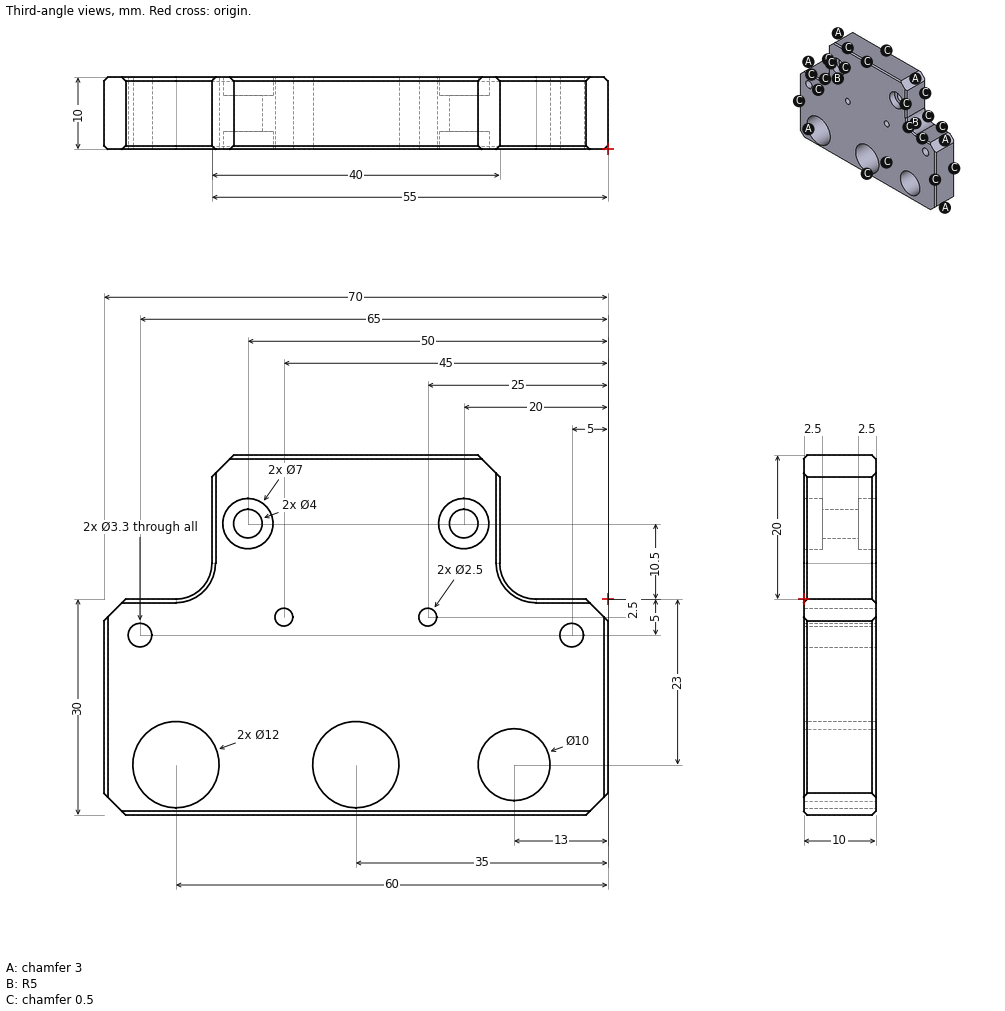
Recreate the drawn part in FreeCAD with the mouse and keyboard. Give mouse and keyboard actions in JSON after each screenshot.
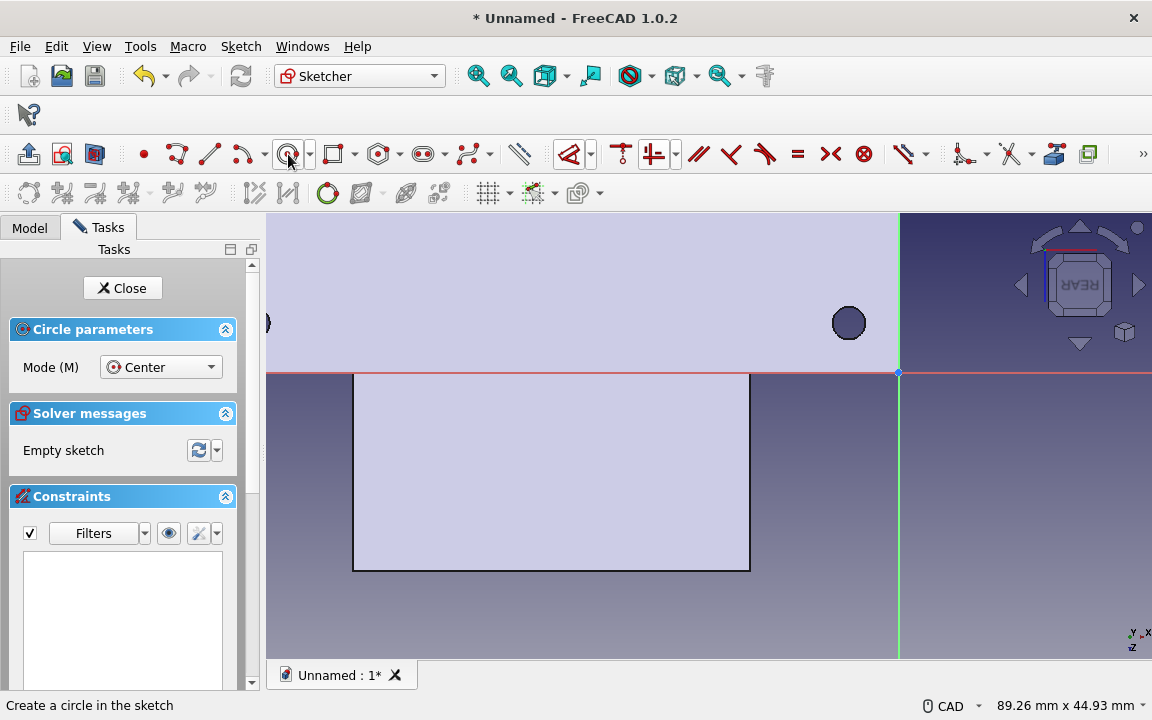
{"action": "left_click", "coordinate": [402, 477]}
{"action": "left_click", "coordinate": [416, 463]}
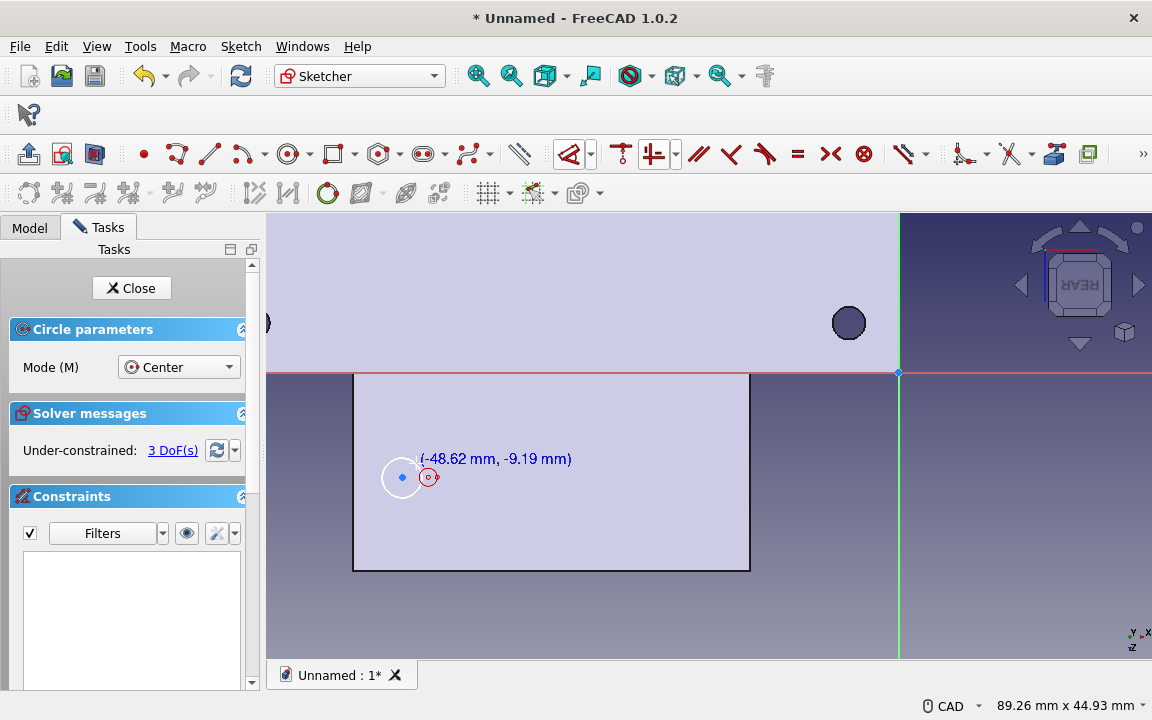
{"action": "left_click", "coordinate": [700, 477]}
{"action": "left_click", "coordinate": [714, 463]}
{"action": "key", "text": "Escape"}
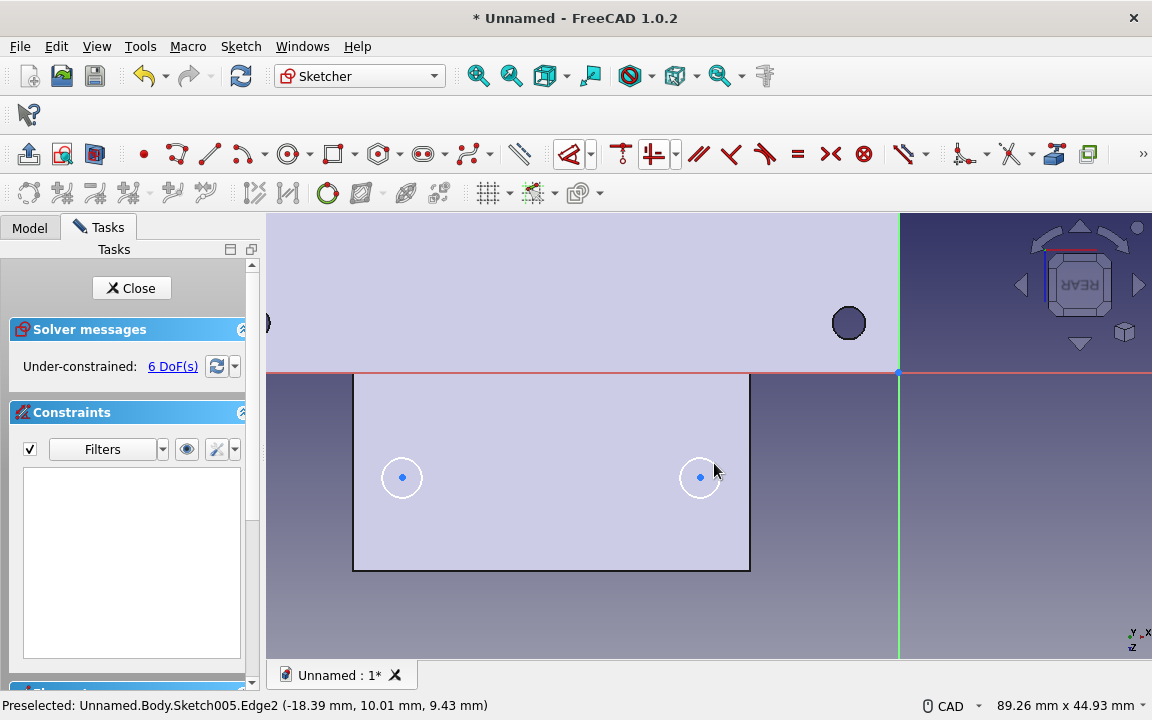
{"action": "left_click", "coordinate": [416, 464]}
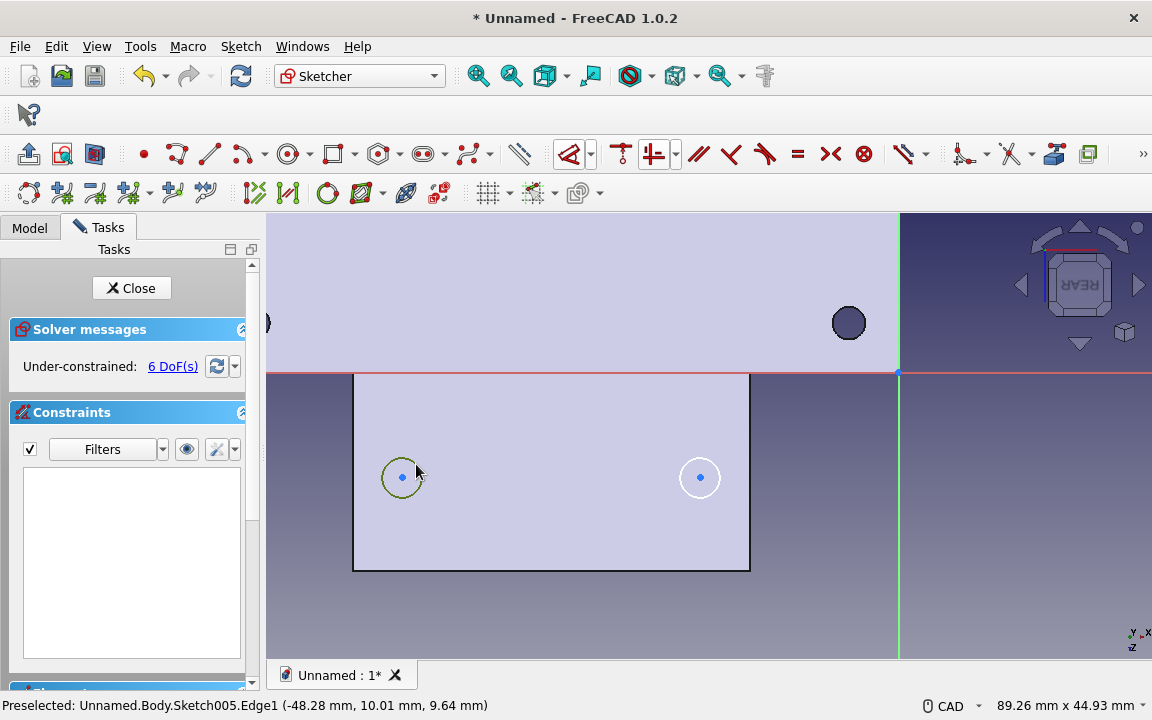
{"action": "left_click", "coordinate": [714, 464]}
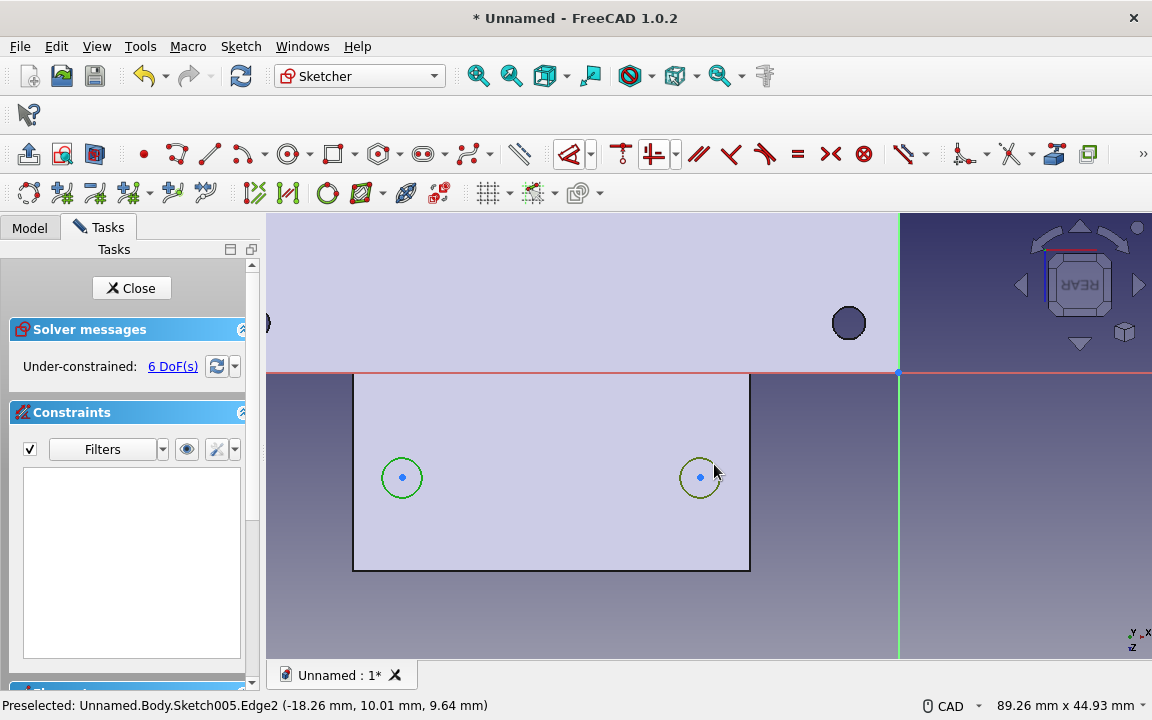
{"action": "left_click", "coordinate": [798, 154]}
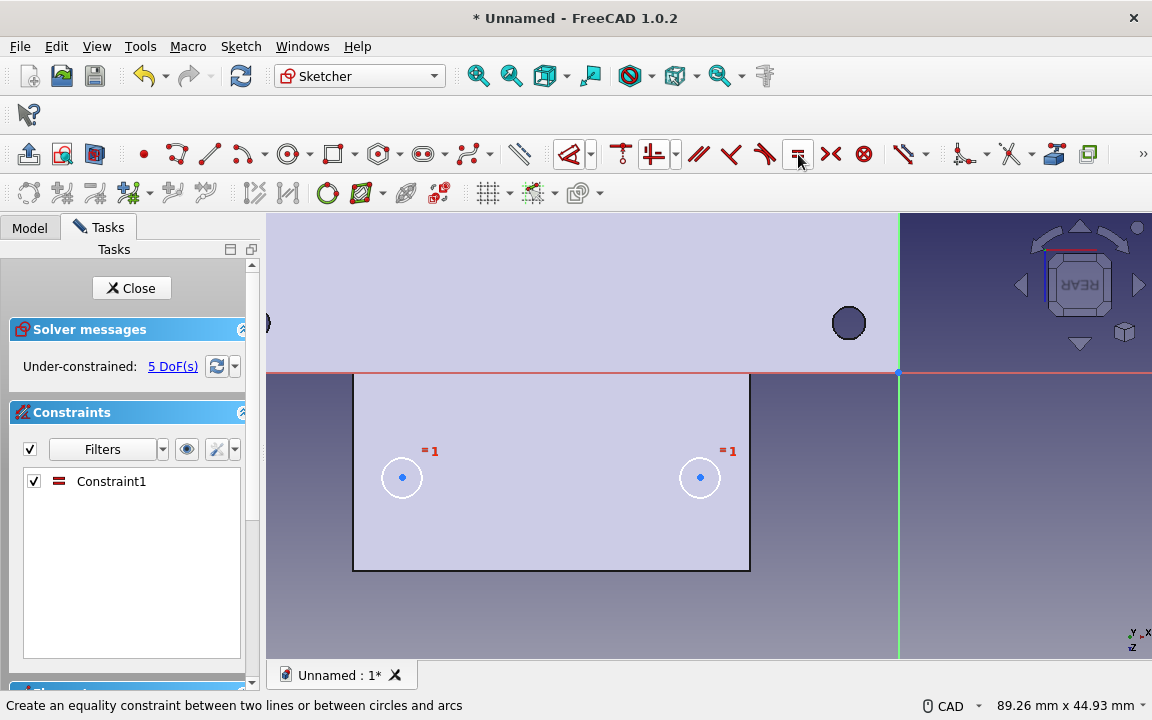
{"action": "left_click", "coordinate": [402, 478]}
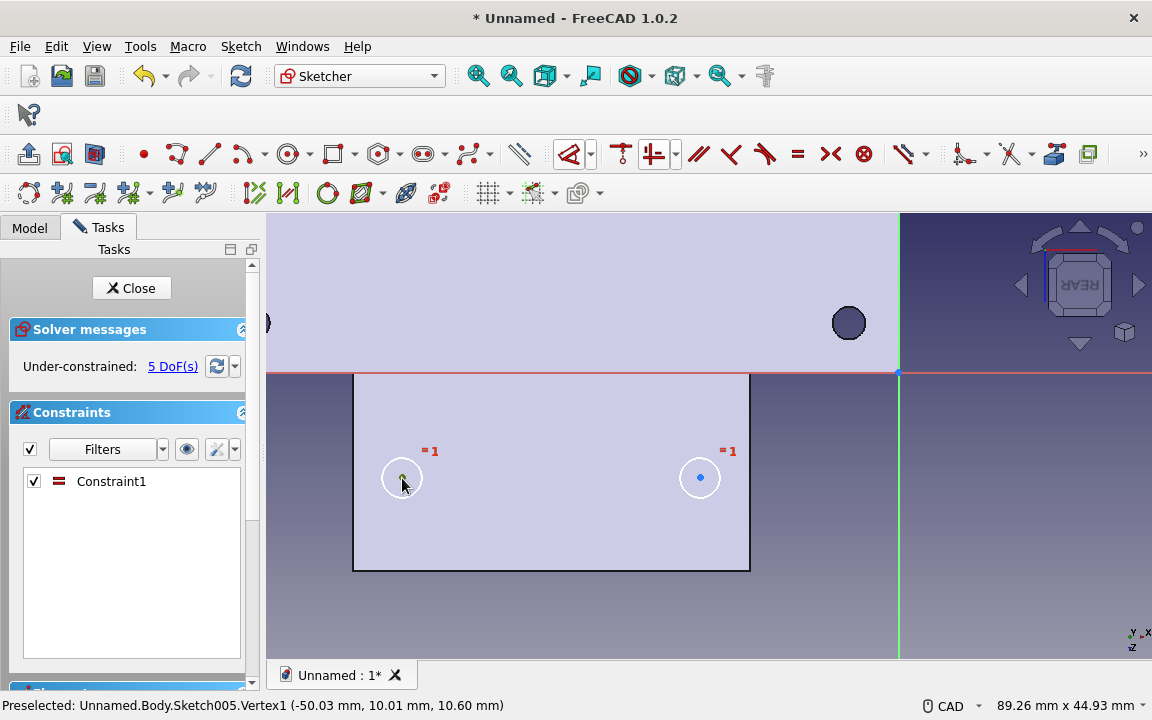
{"action": "left_click", "coordinate": [700, 478]}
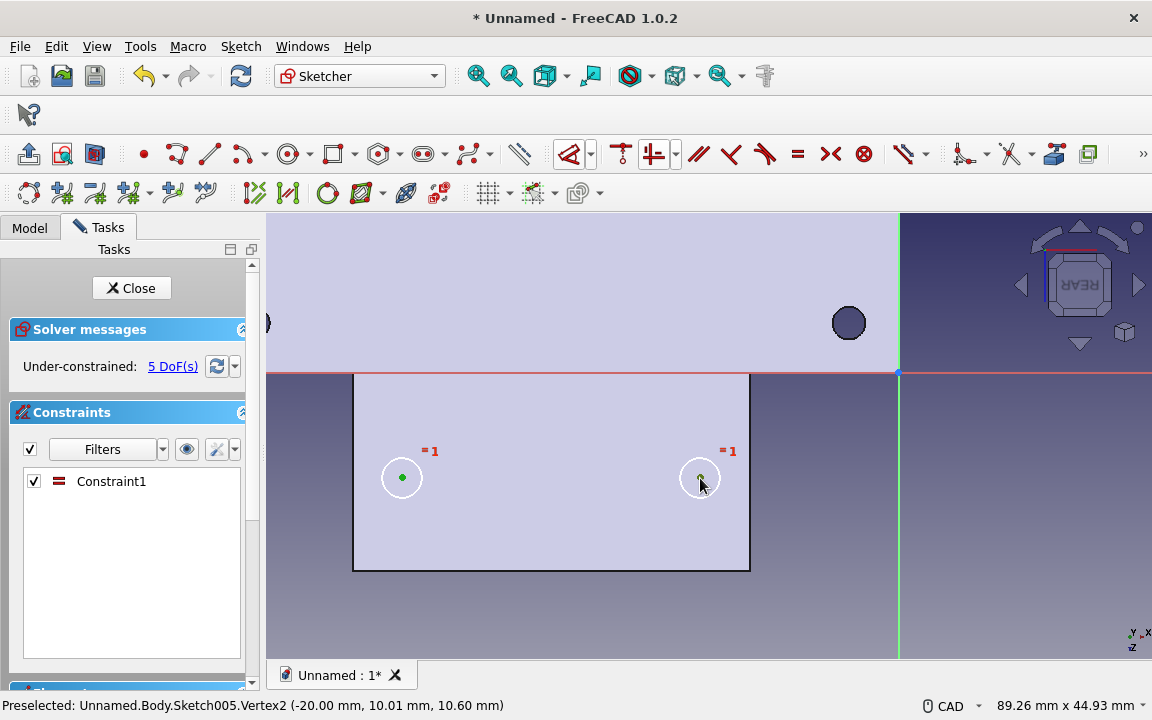
{"action": "left_click", "coordinate": [676, 154]}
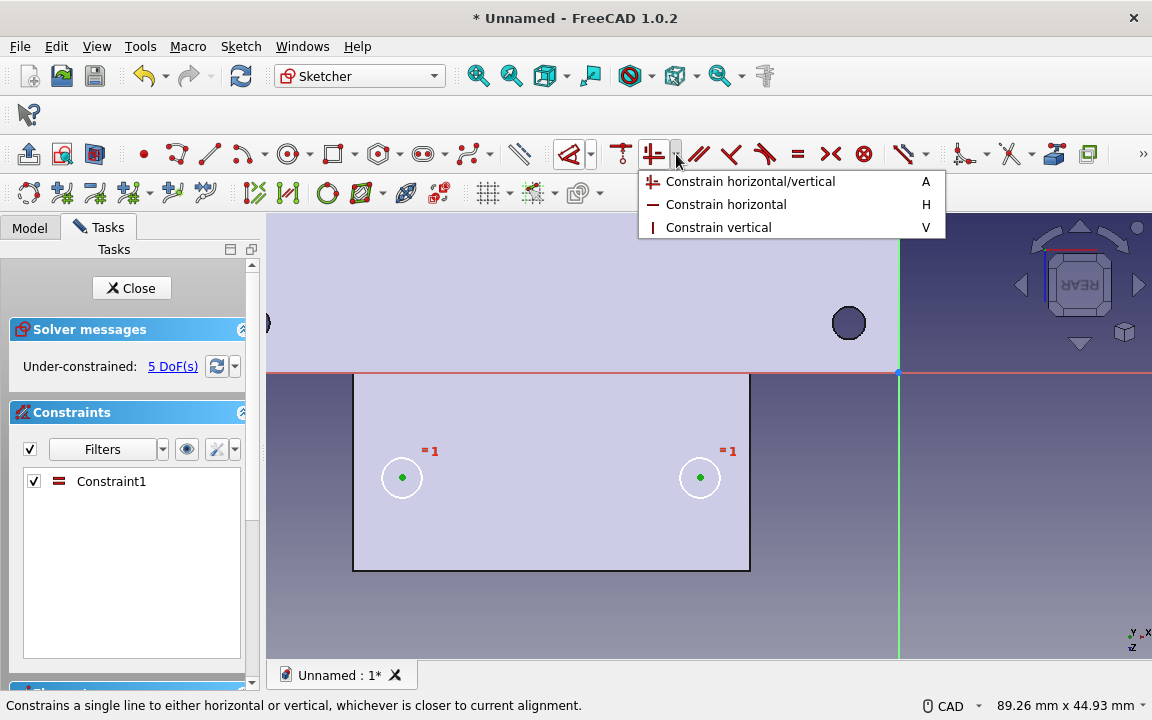
{"action": "left_click", "coordinate": [792, 204]}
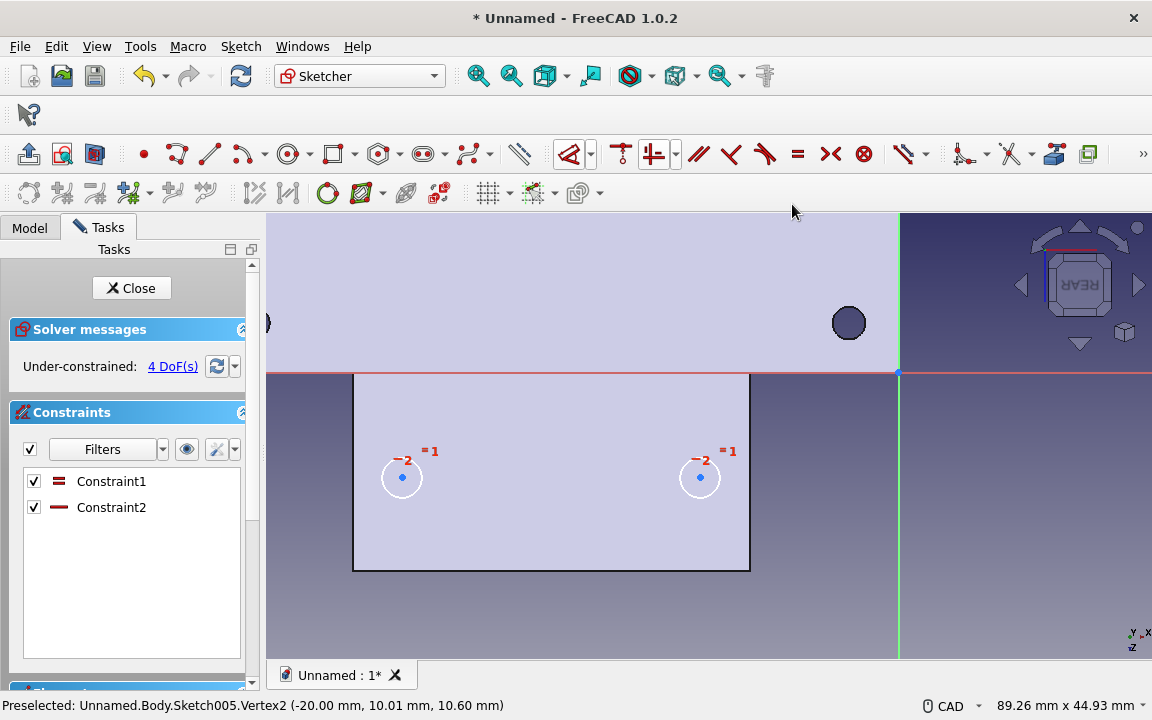
{"action": "left_click", "coordinate": [416, 464]}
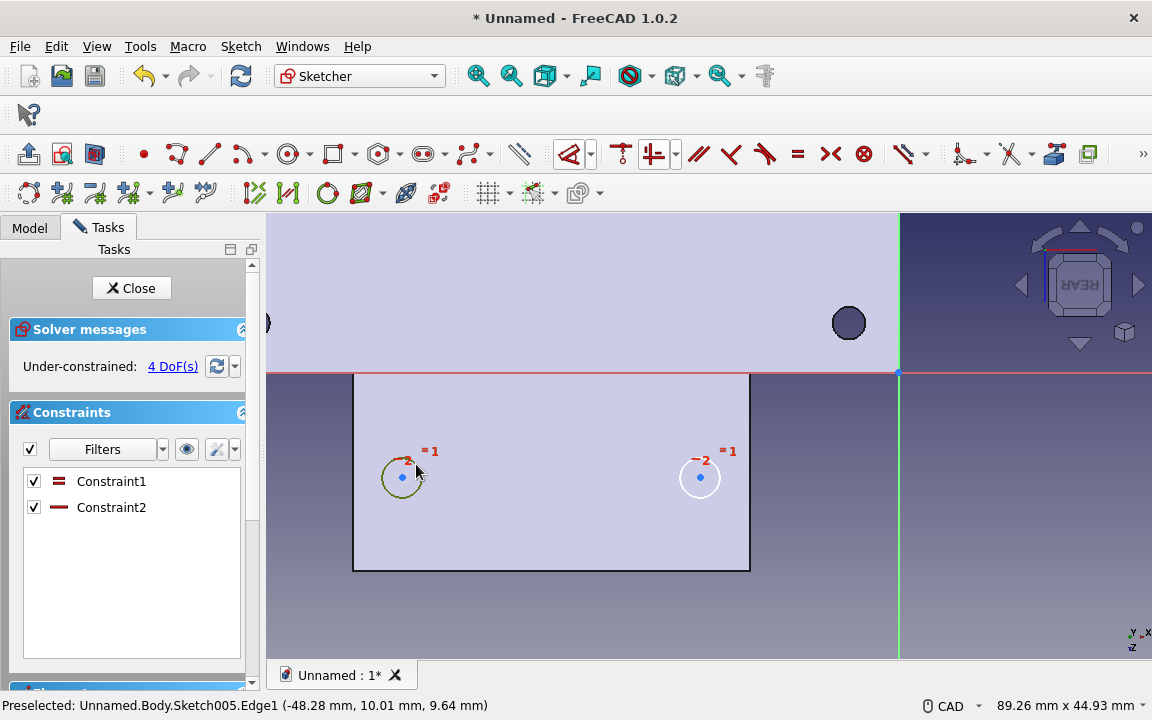
{"action": "left_click", "coordinate": [590, 154]}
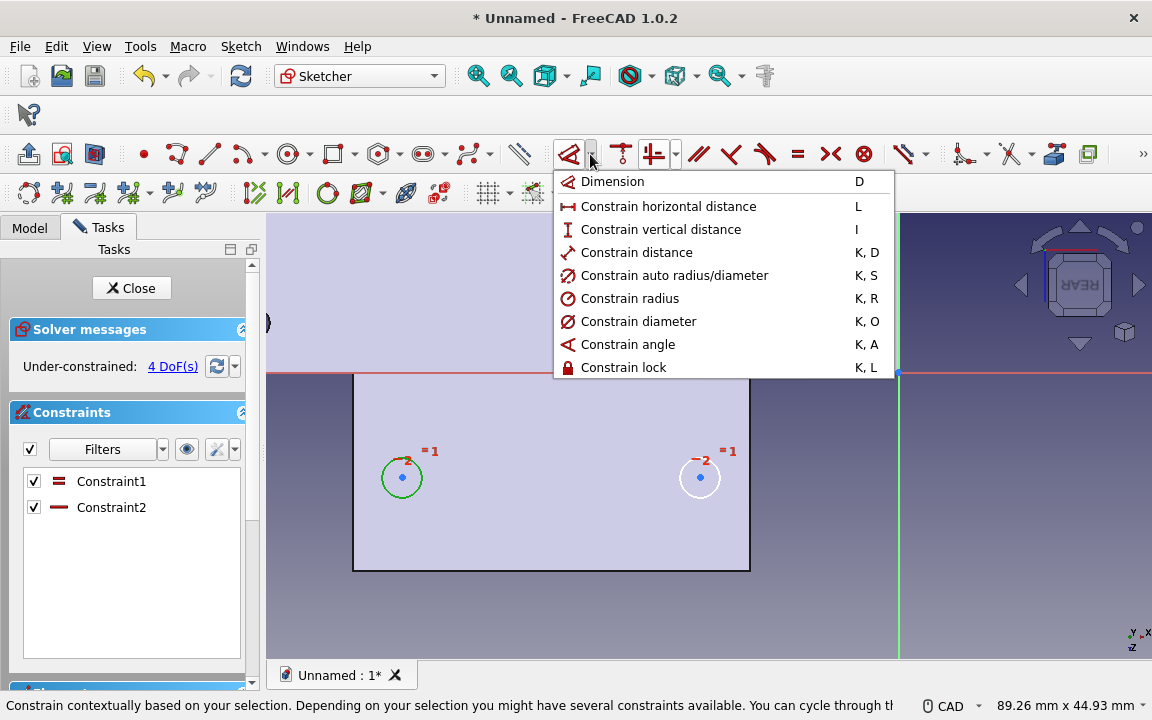
{"action": "left_click", "coordinate": [724, 322]}